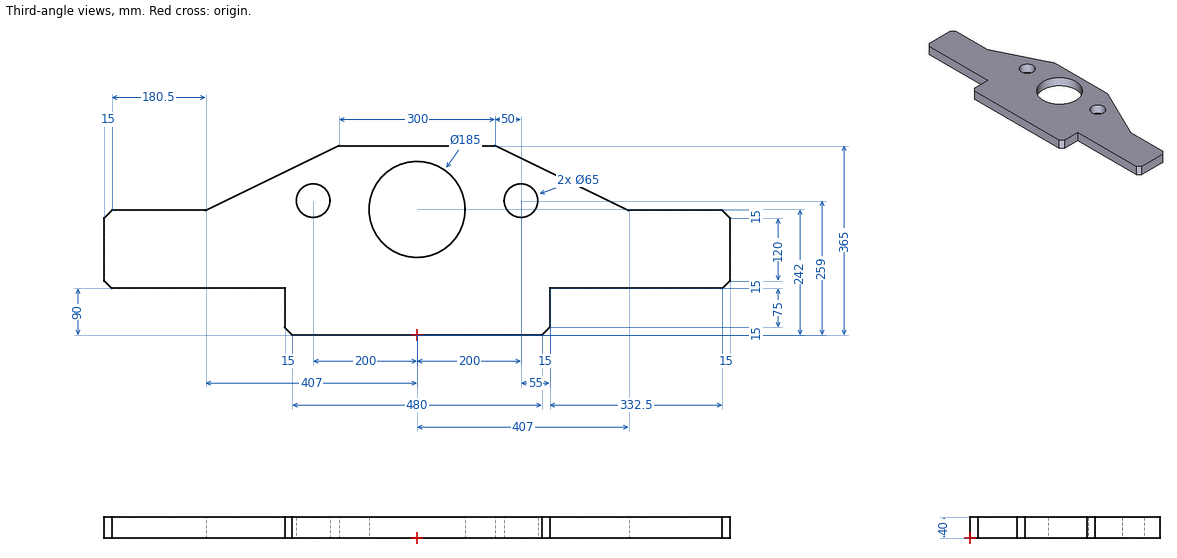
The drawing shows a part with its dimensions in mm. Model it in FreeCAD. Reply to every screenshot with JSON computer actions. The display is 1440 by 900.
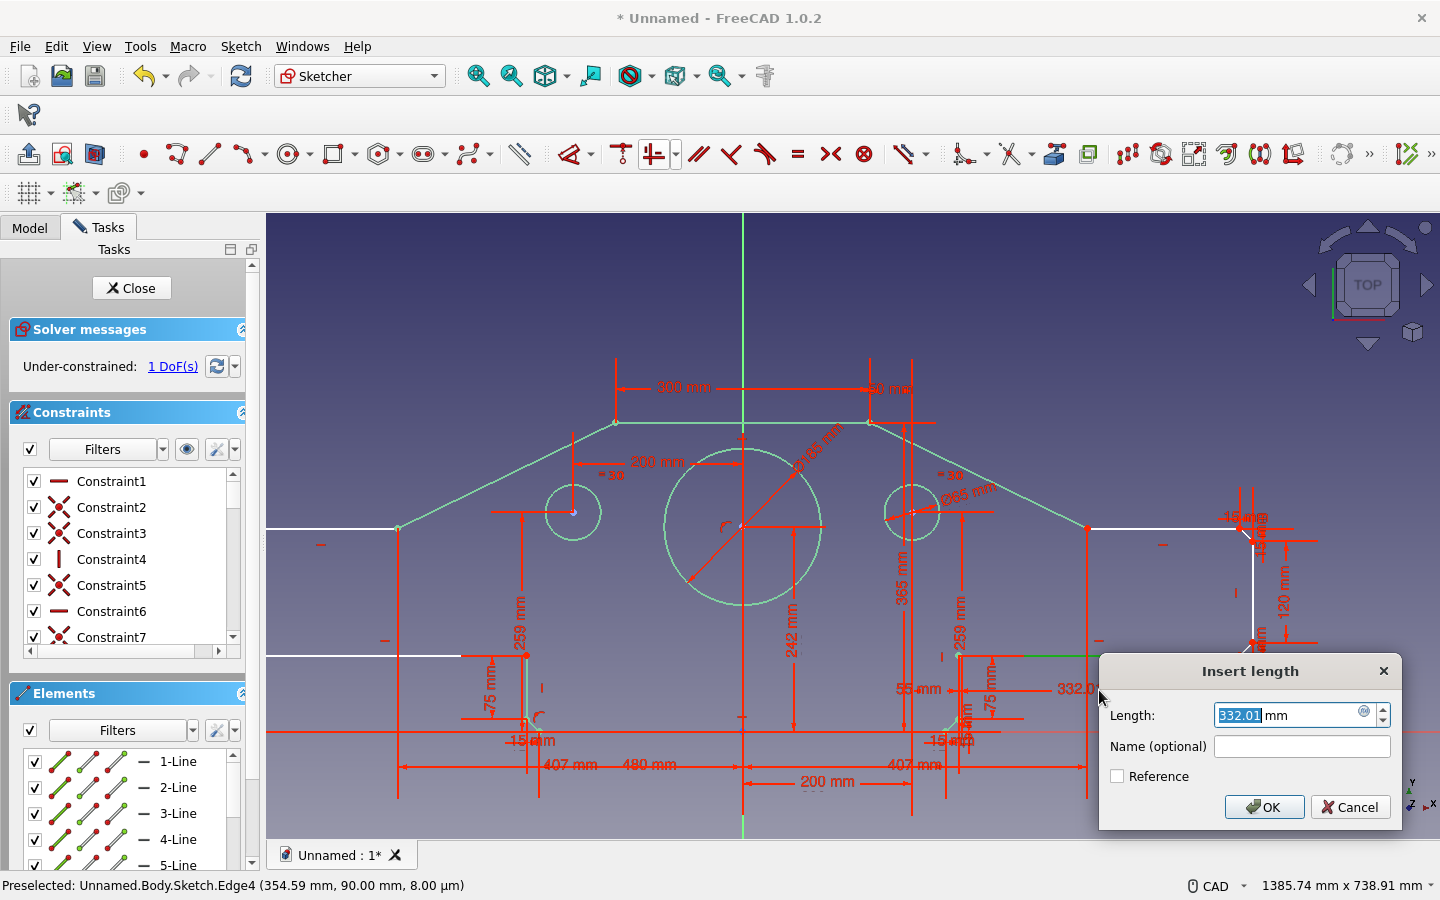
{"action": "type", "text": "332.5"}
{"action": "key", "text": "Return"}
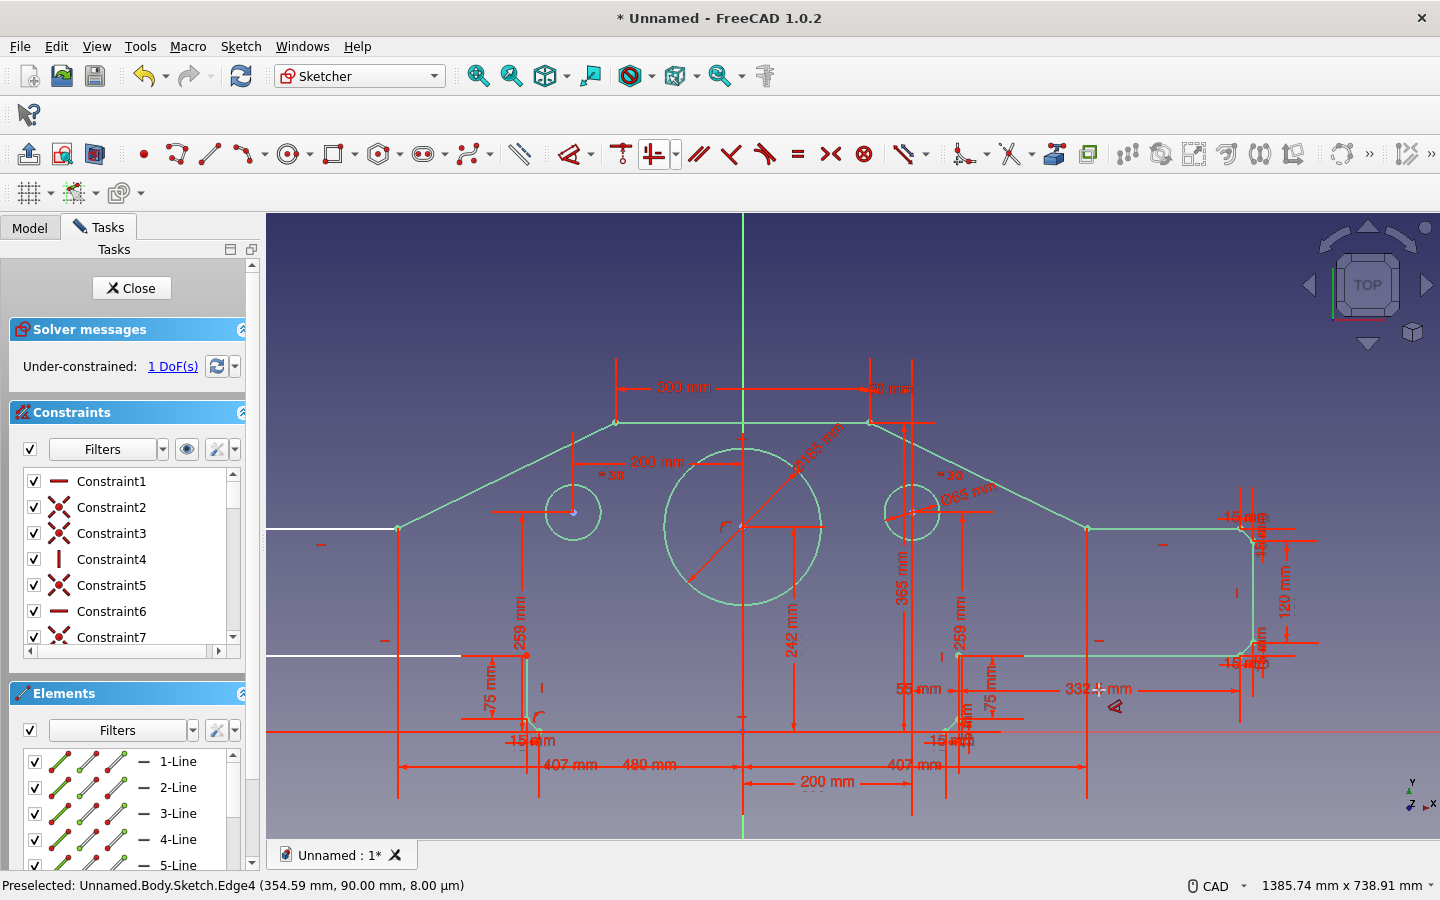
{"action": "left_click", "coordinate": [352, 529]}
{"action": "left_click", "coordinate": [346, 495]}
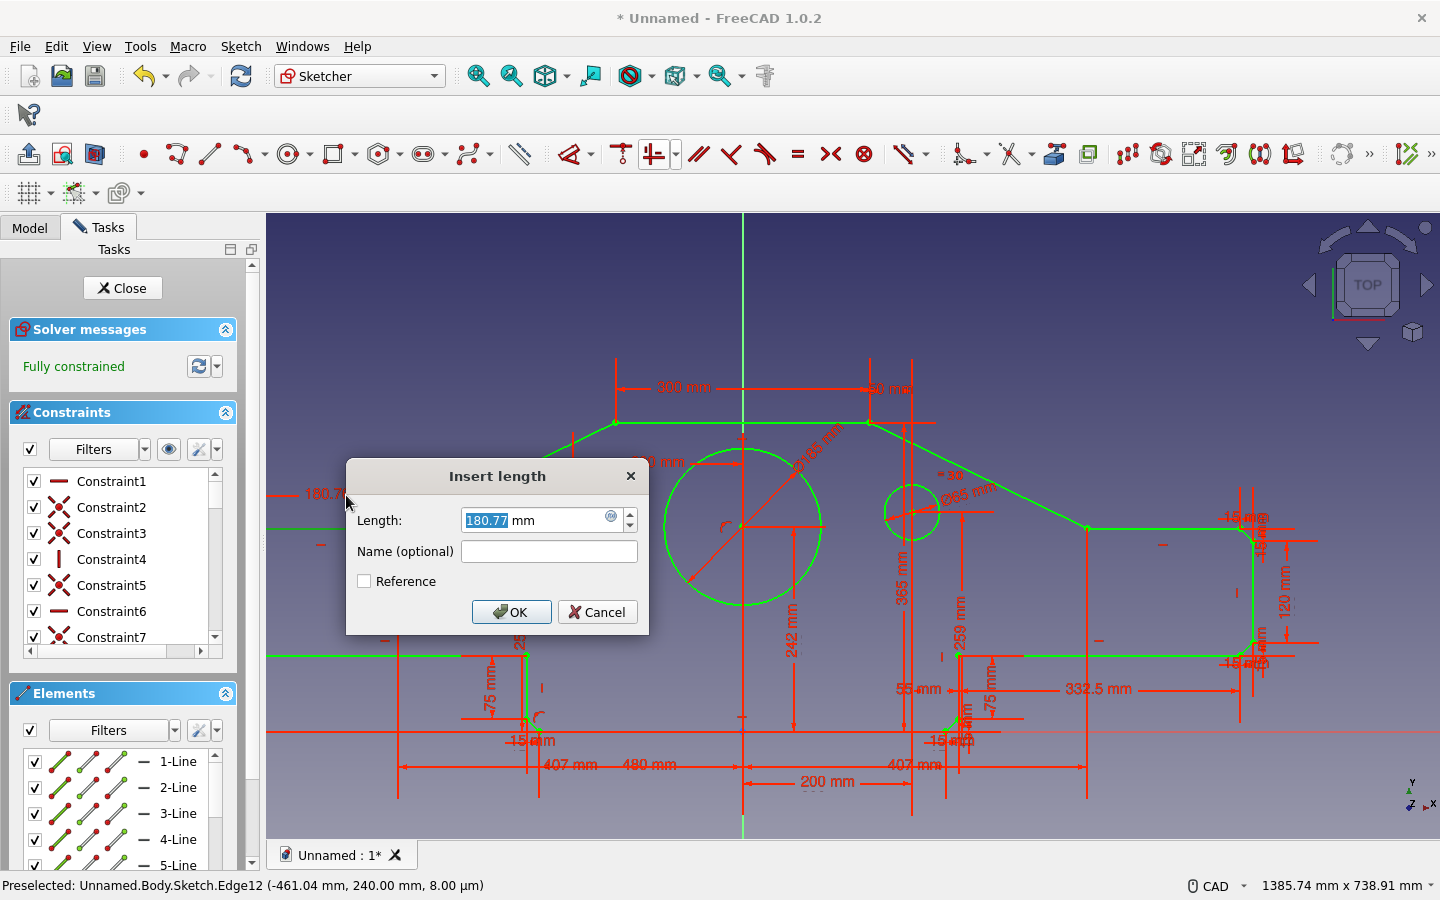
{"action": "type", "text": "180.5"}
{"action": "key", "text": "Return"}
{"action": "key", "text": "Escape"}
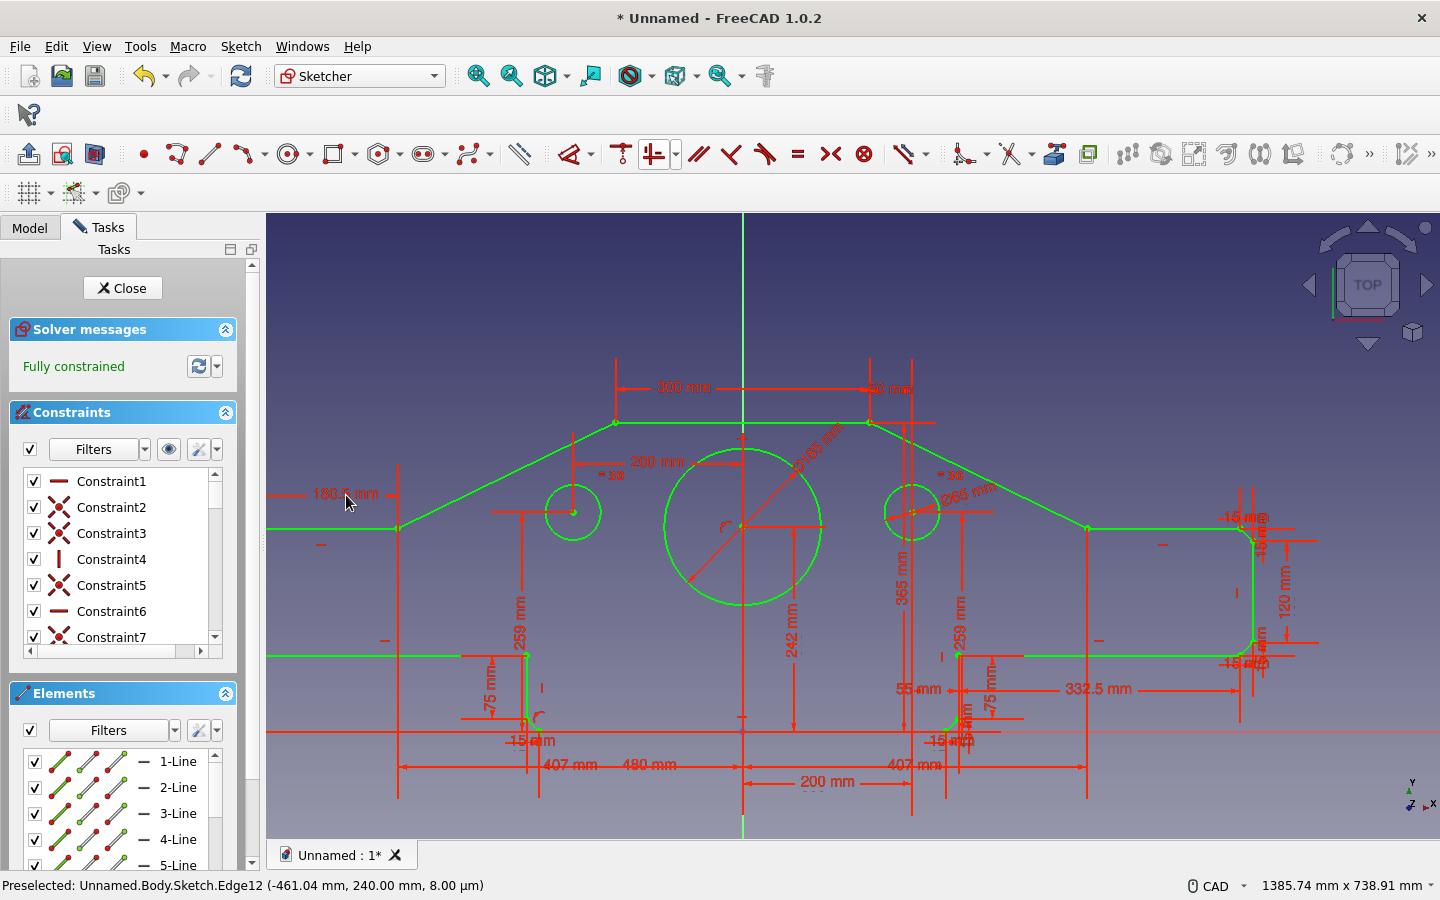
{"action": "left_click", "coordinate": [123, 288]}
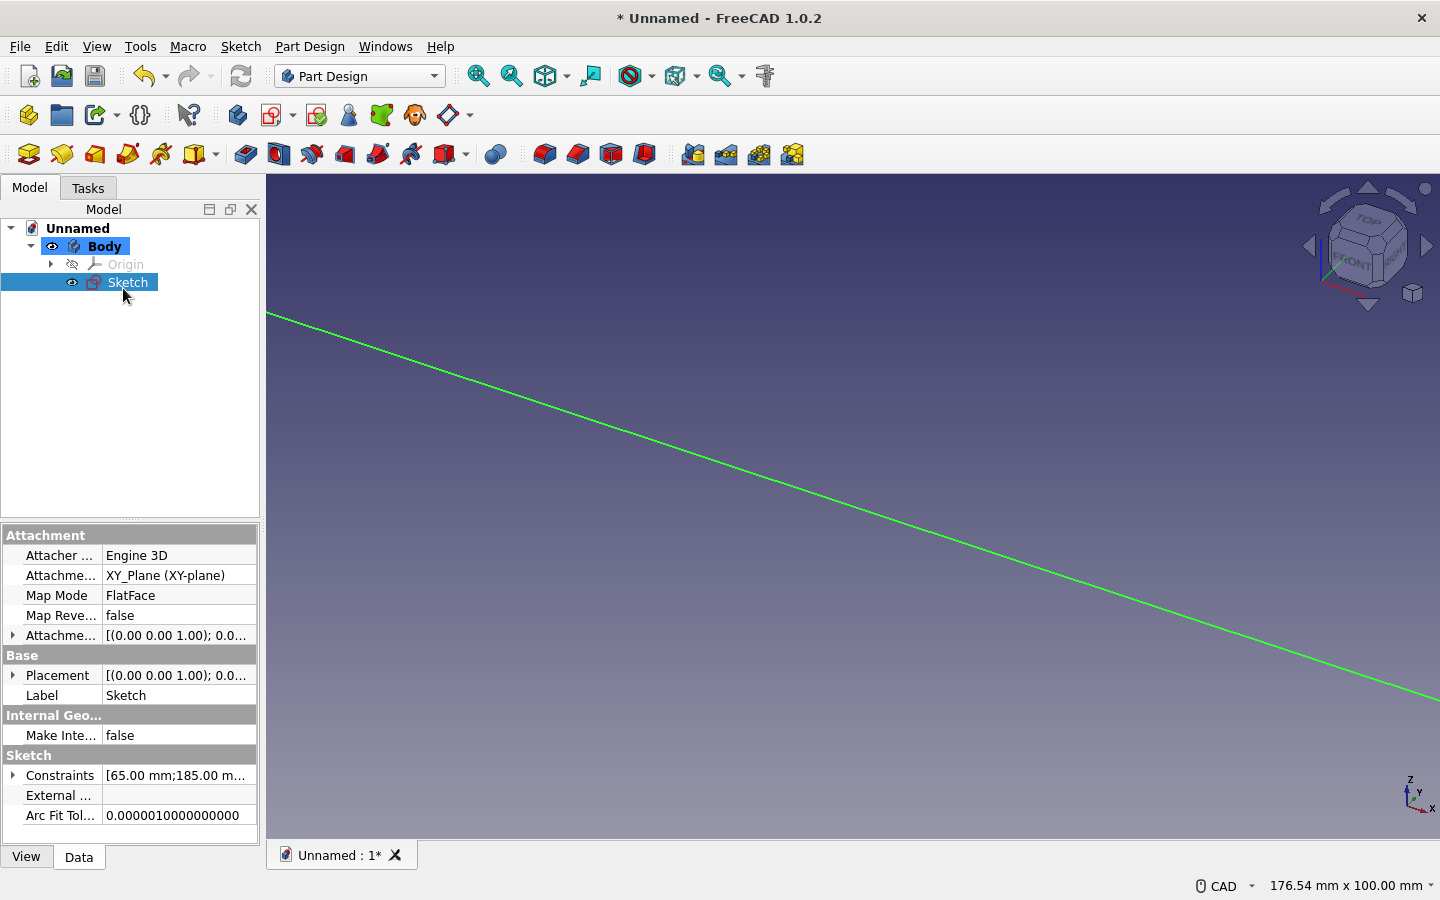
{"action": "left_click", "coordinate": [29, 154]}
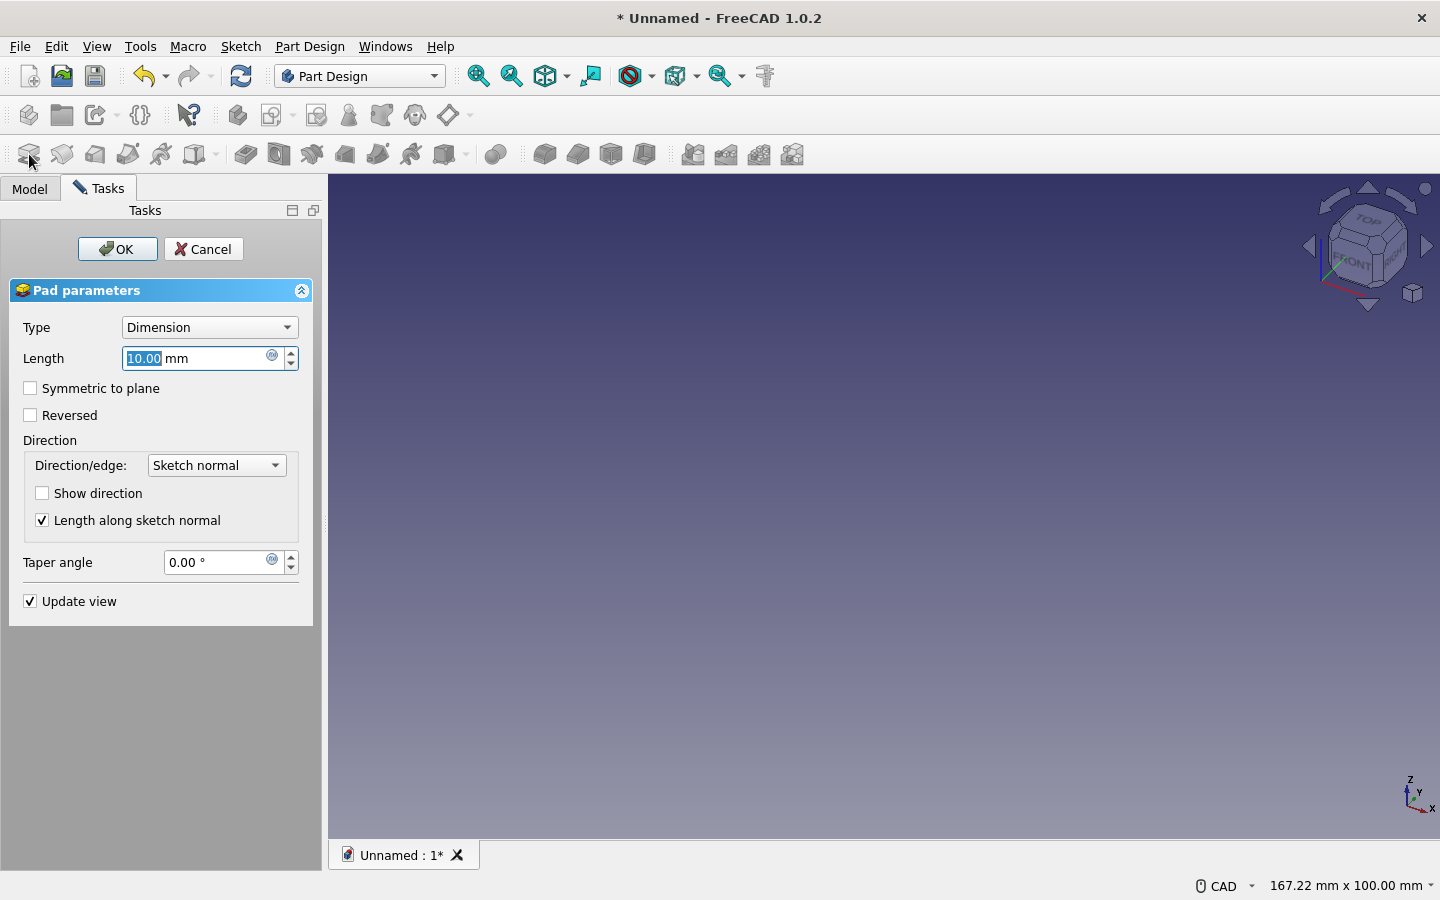
{"action": "type", "text": "40"}
{"action": "key", "text": "Tab"}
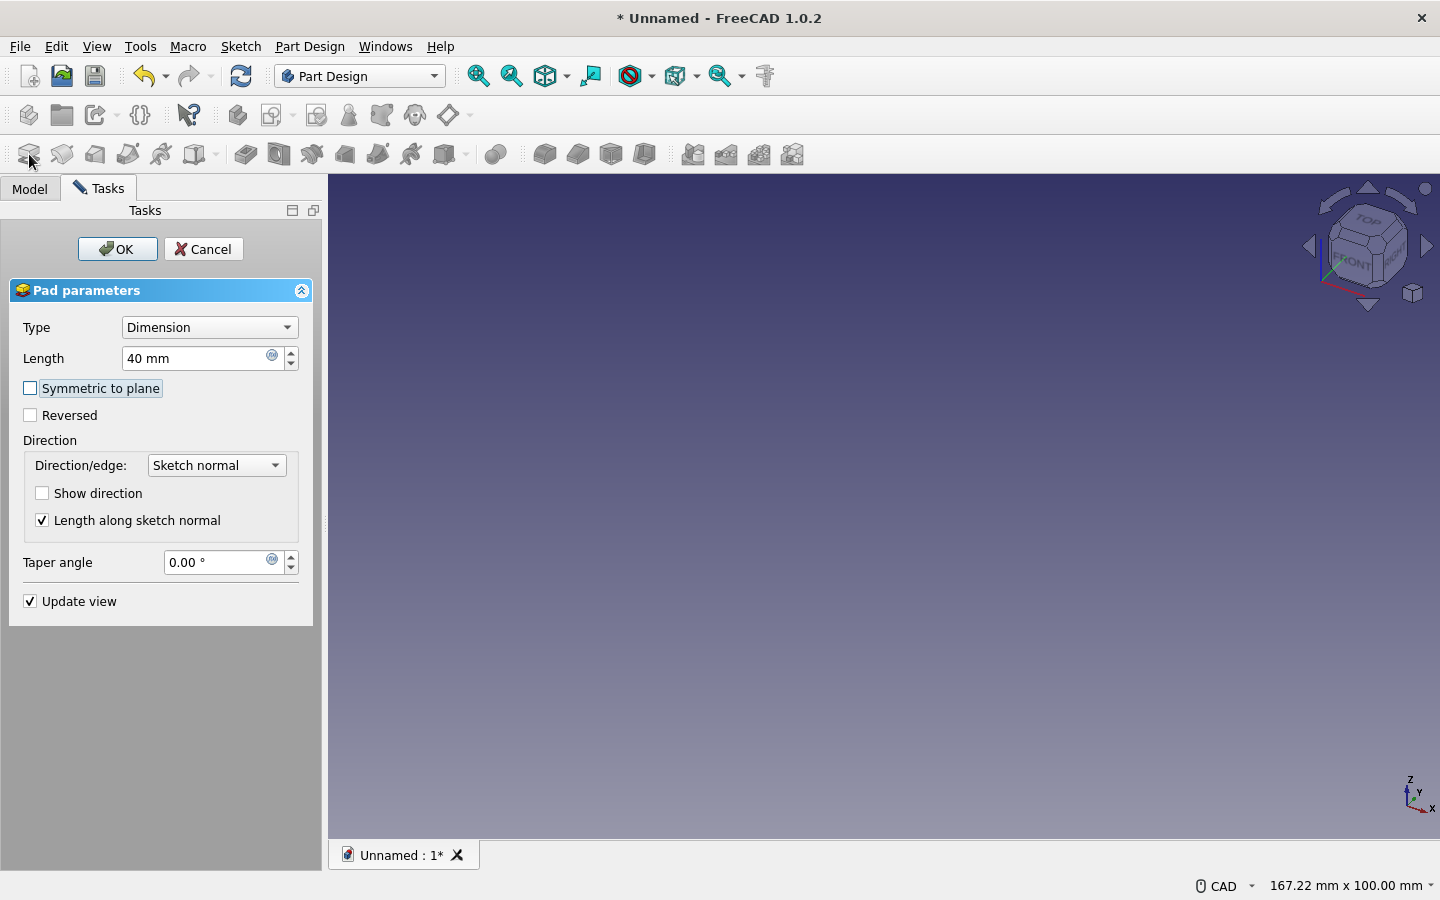
{"action": "left_click", "coordinate": [118, 249]}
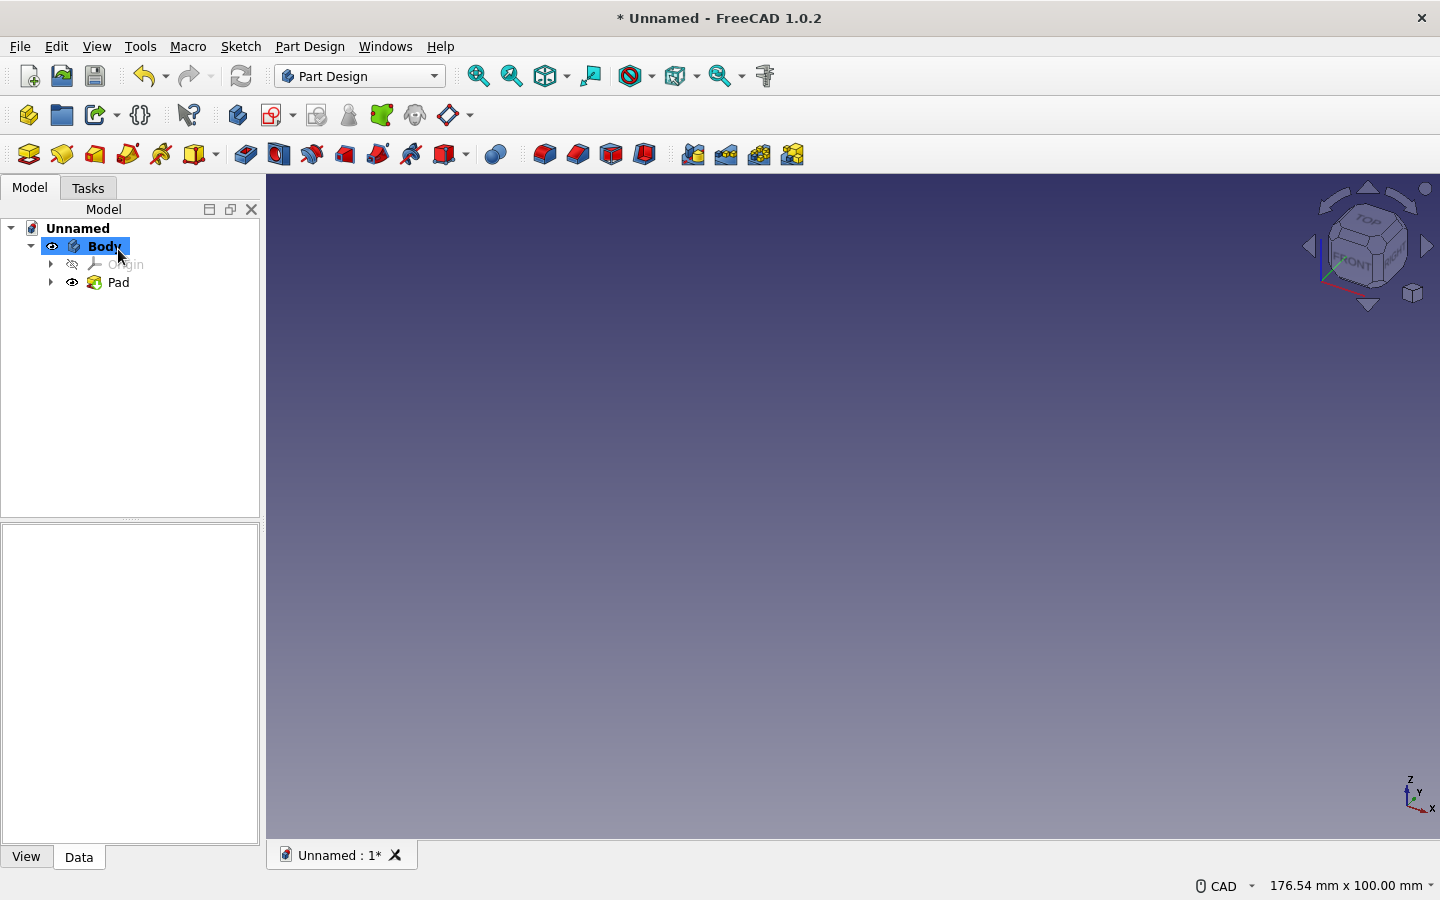
{"action": "key", "text": "0"}